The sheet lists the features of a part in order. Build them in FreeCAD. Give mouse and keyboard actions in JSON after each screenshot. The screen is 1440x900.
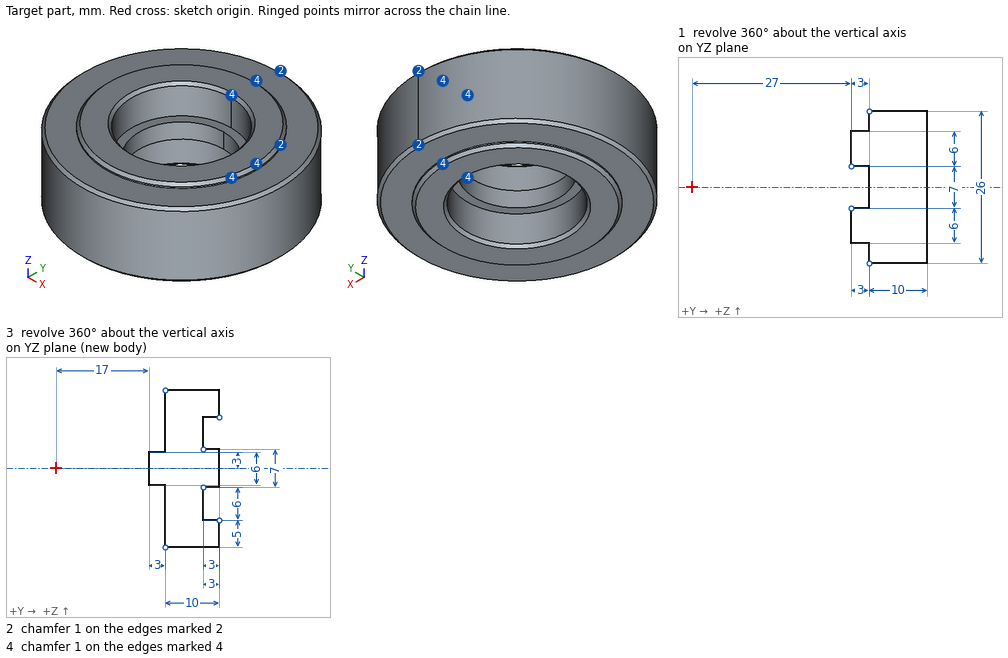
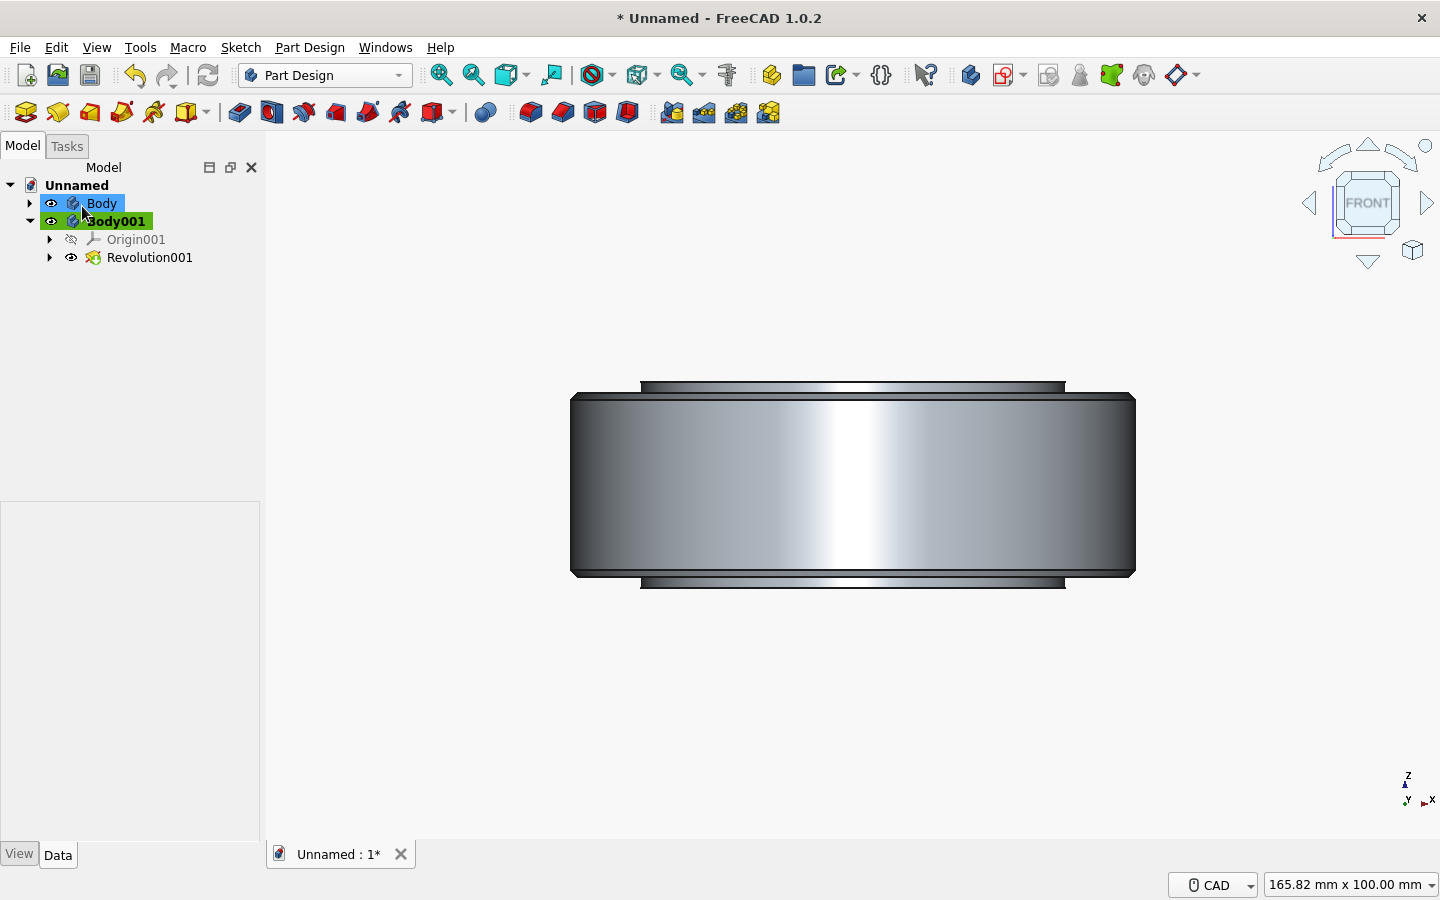
{"action": "left_click", "coordinate": [442, 76]}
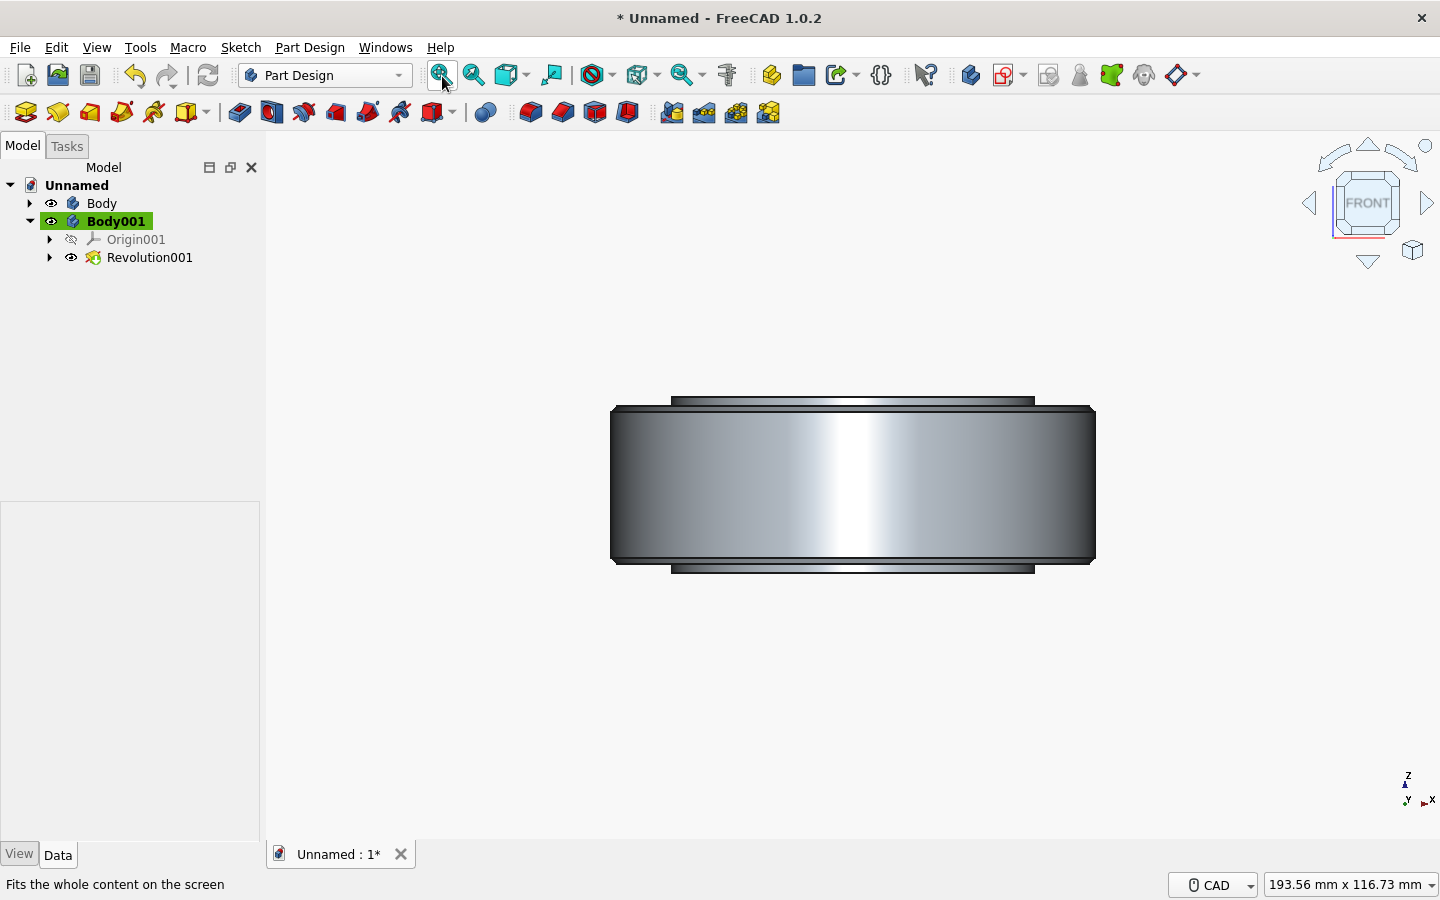
{"action": "left_click", "coordinate": [853, 572]}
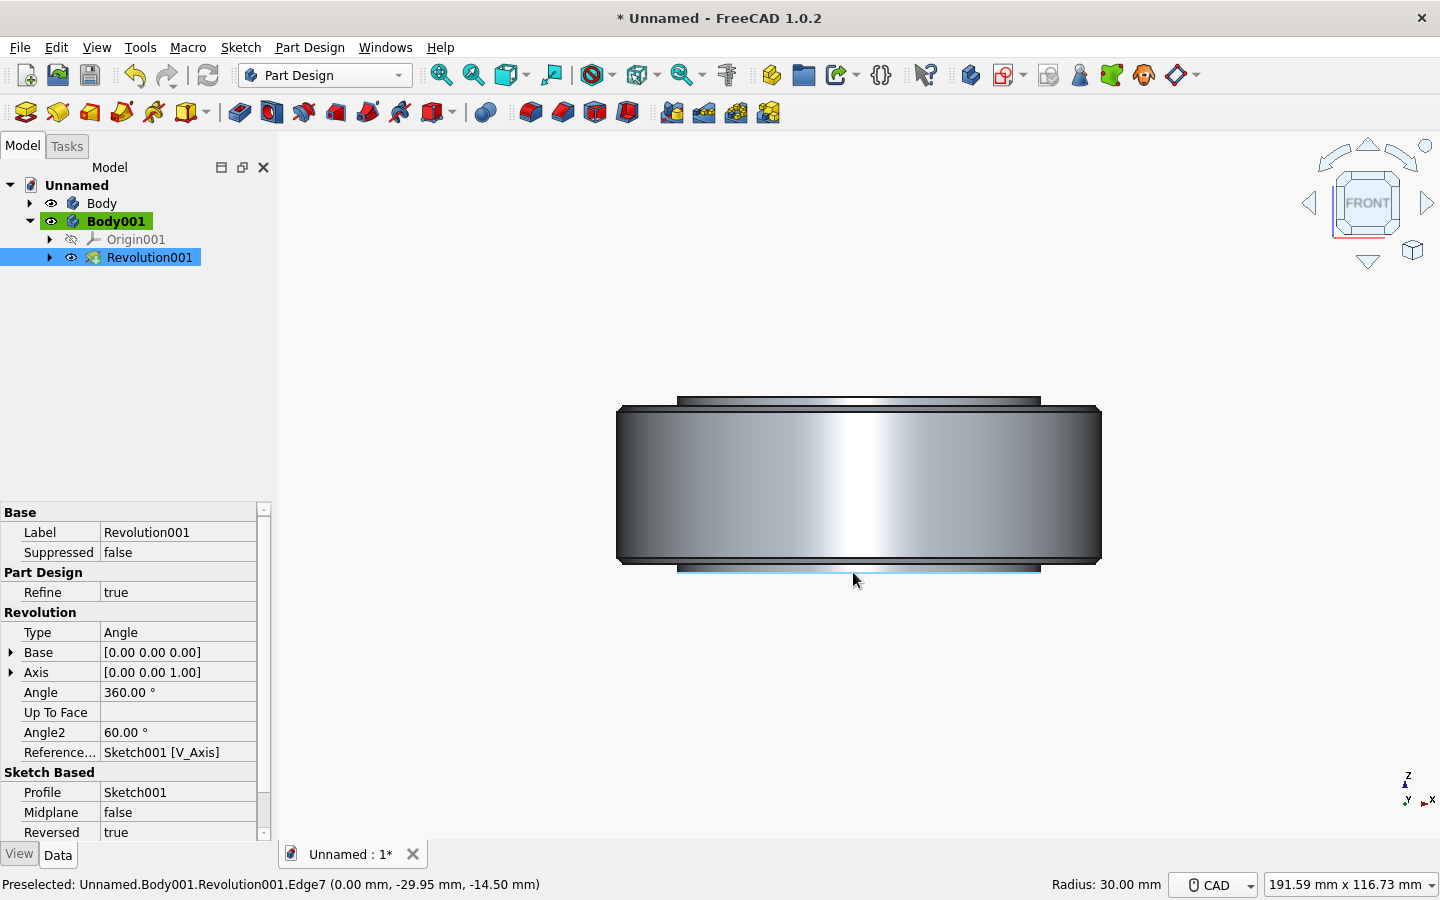
{"action": "left_click", "coordinate": [859, 396], "text": "ctrl"}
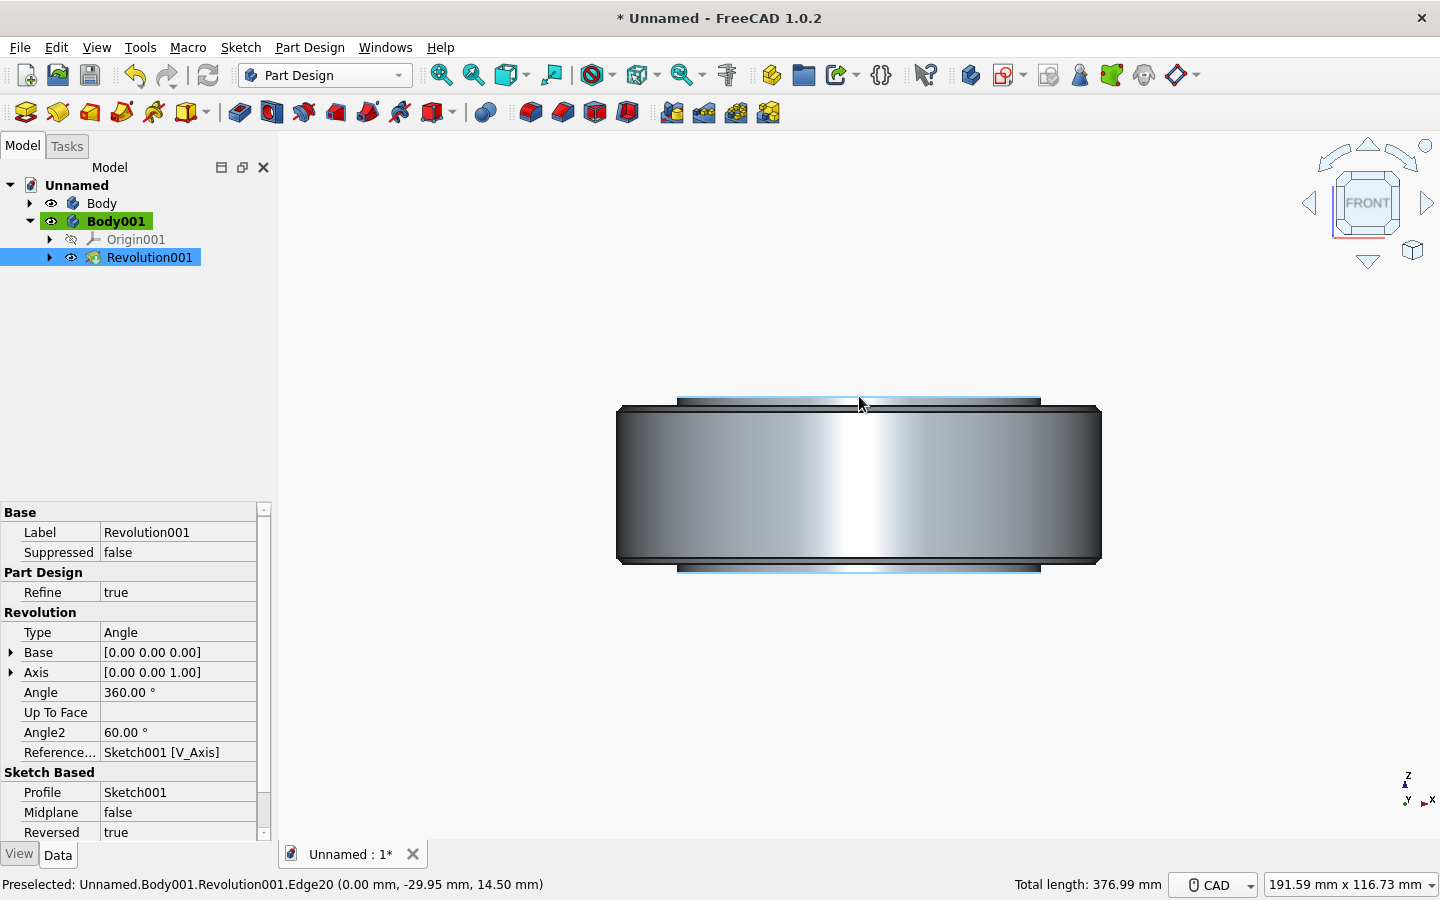
{"action": "key", "text": "0"}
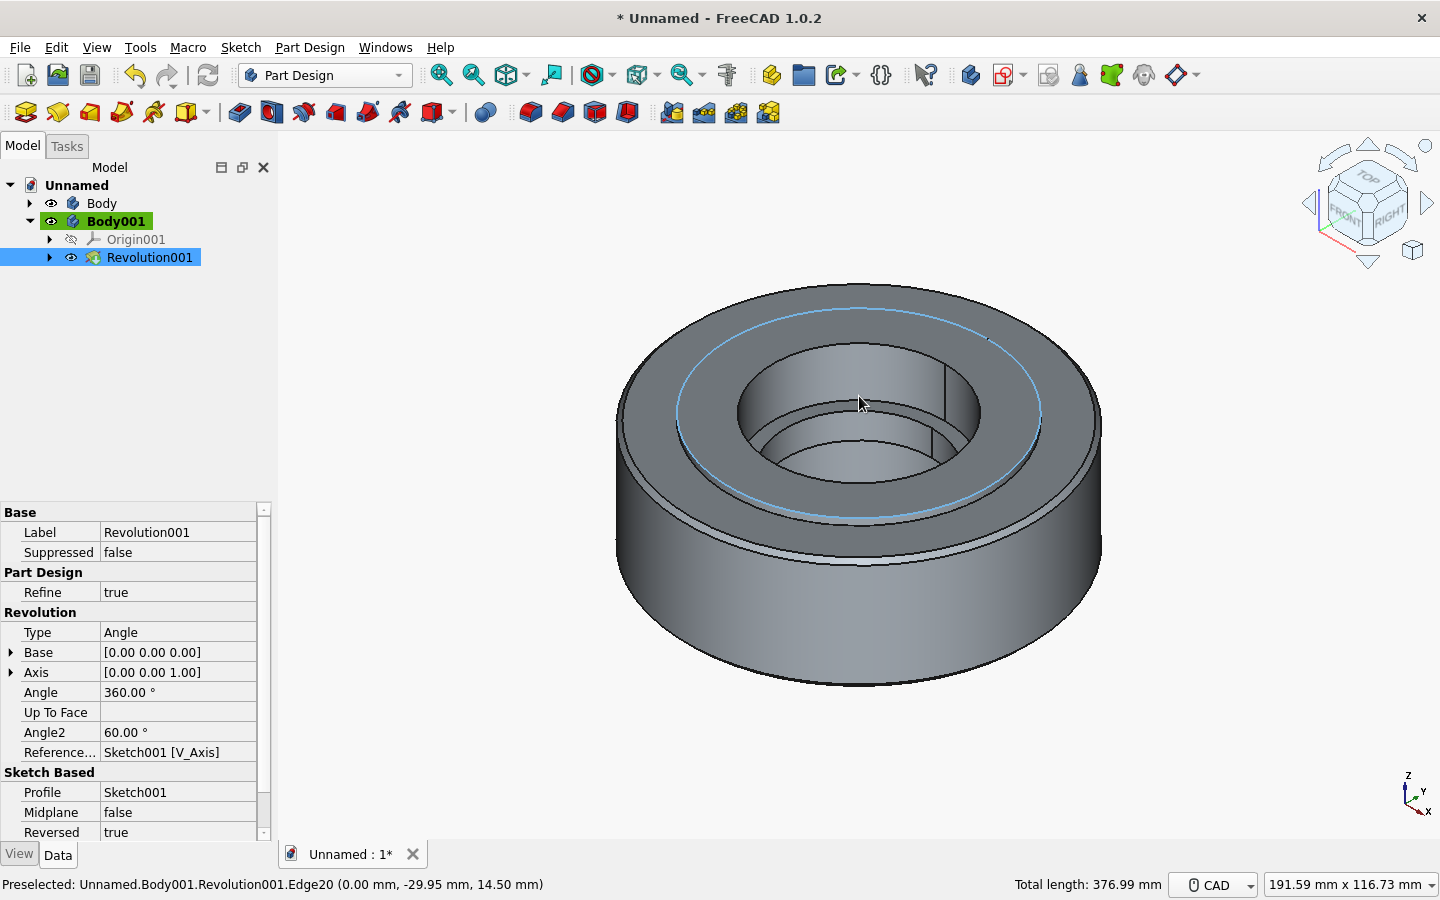
{"action": "left_click", "coordinate": [751, 380], "text": "ctrl"}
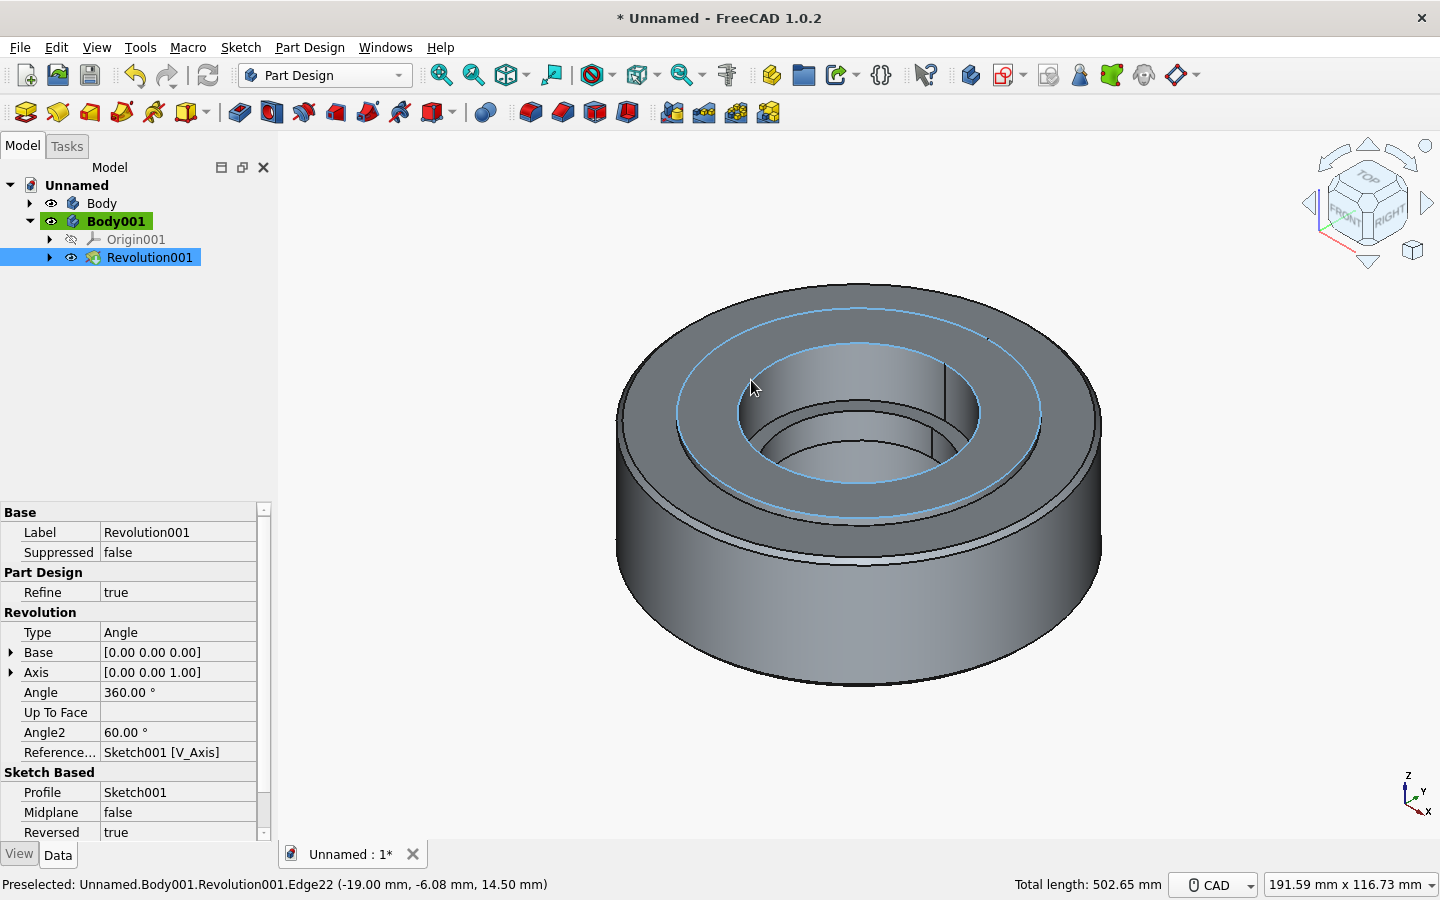
{"action": "key", "text": "2"}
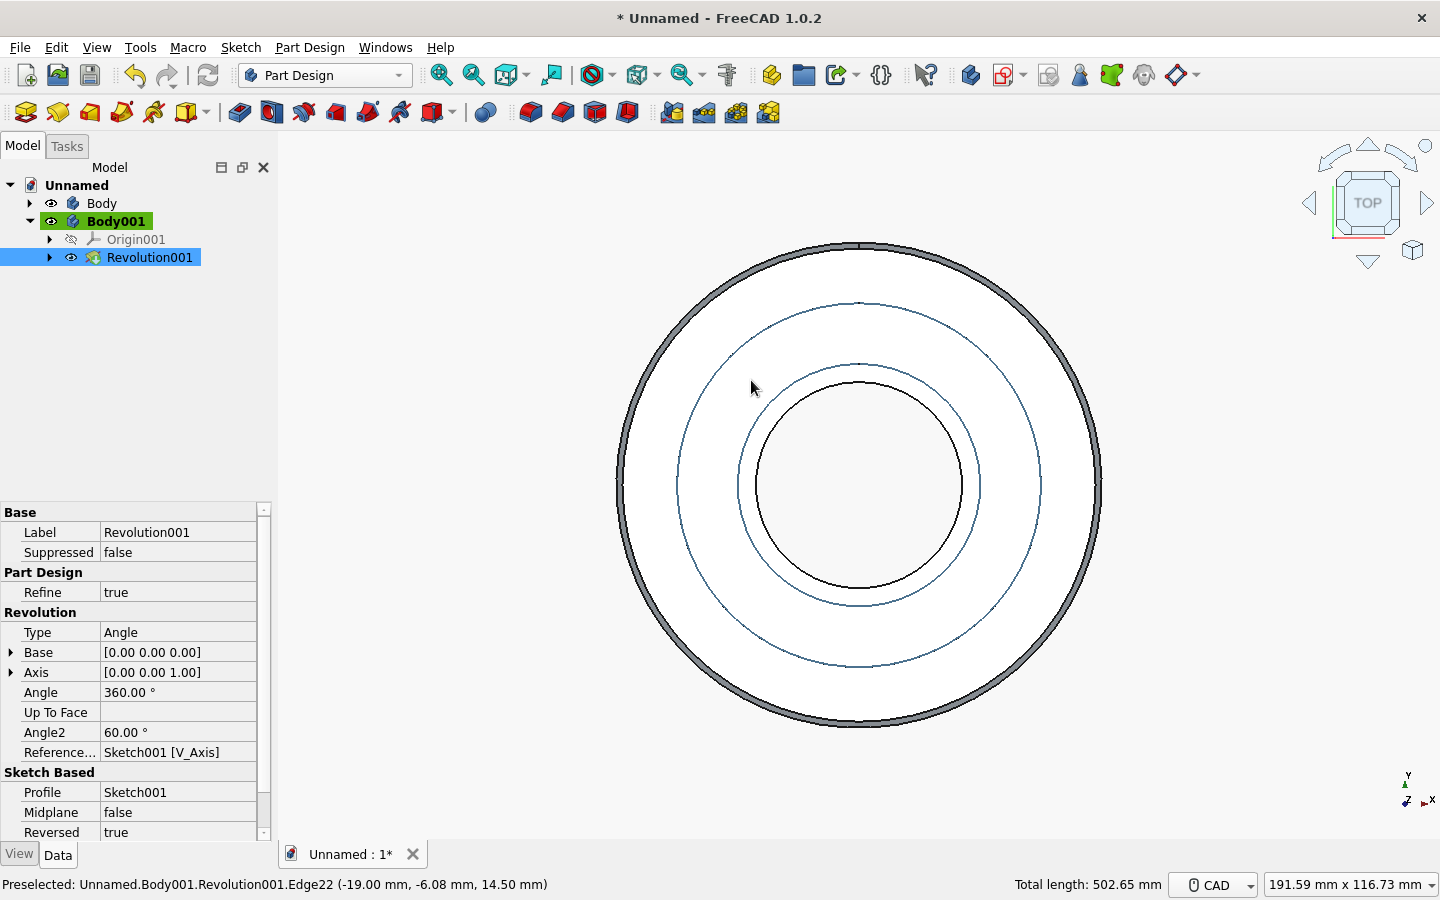
{"action": "key", "text": "1"}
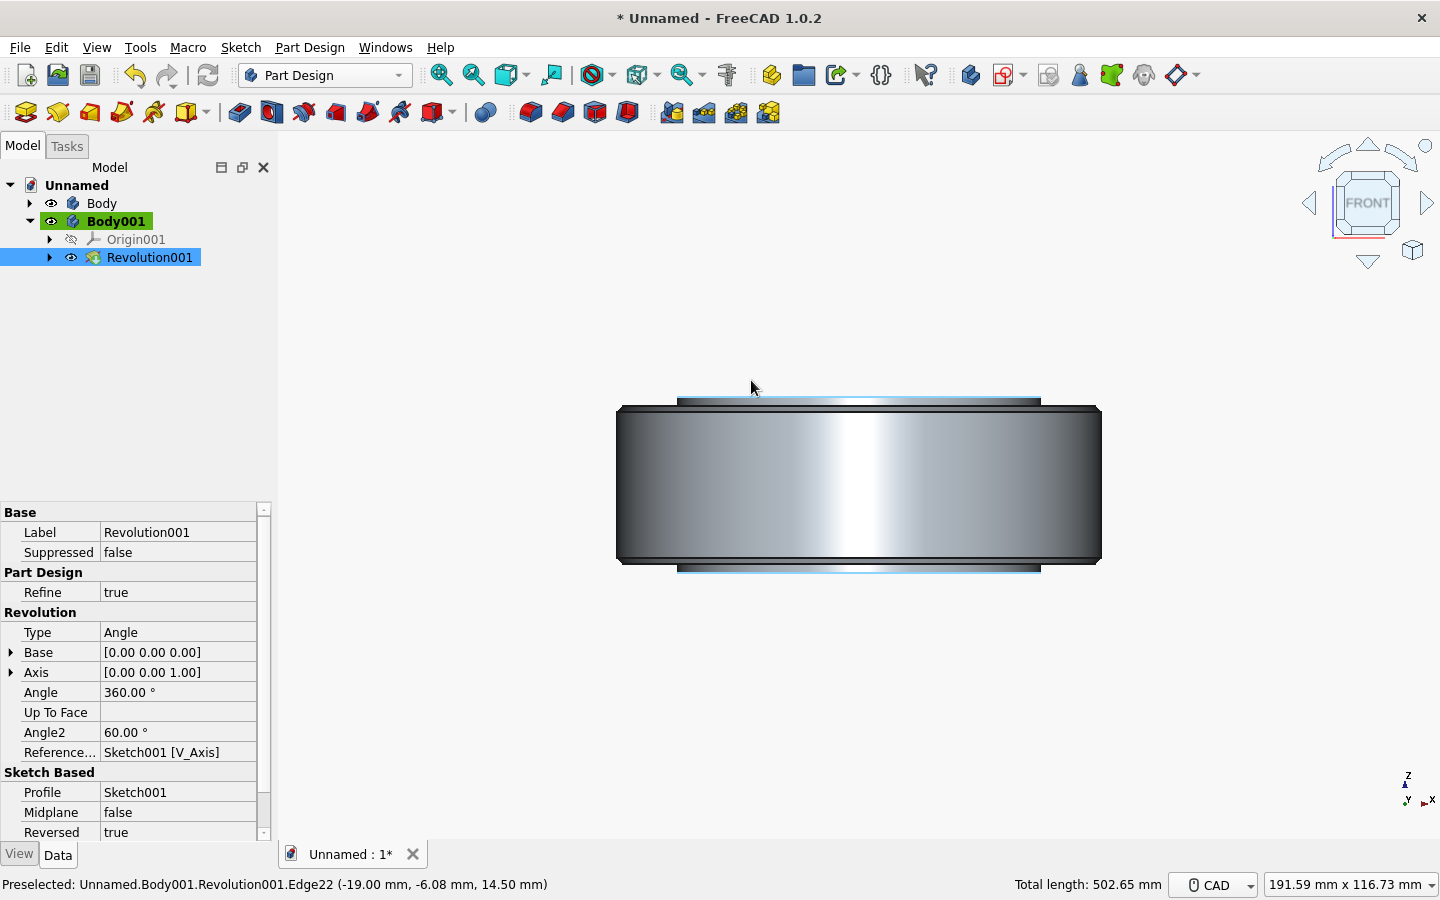
{"action": "left_click", "coordinate": [442, 76]}